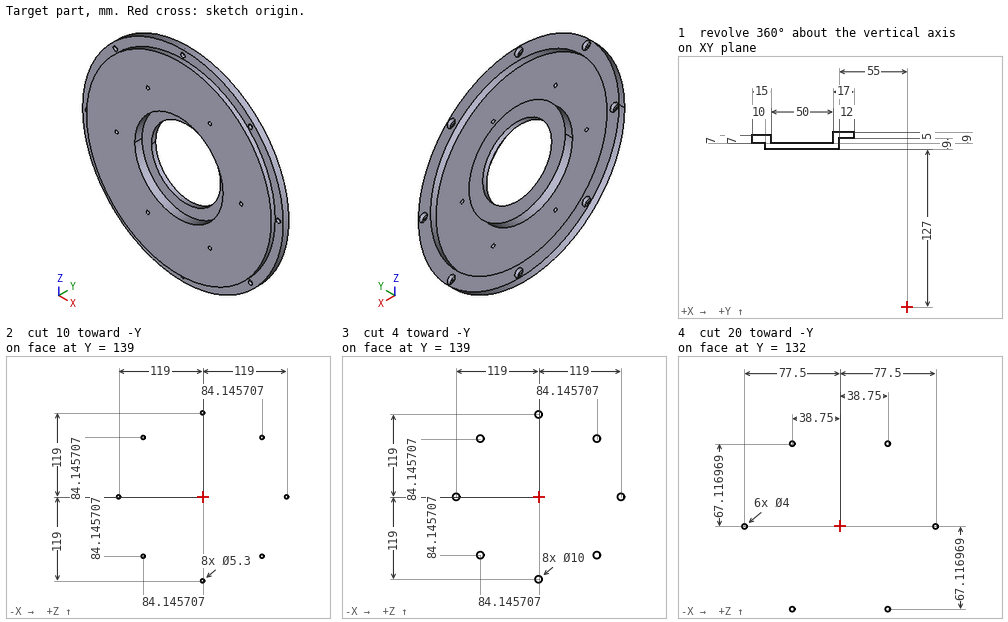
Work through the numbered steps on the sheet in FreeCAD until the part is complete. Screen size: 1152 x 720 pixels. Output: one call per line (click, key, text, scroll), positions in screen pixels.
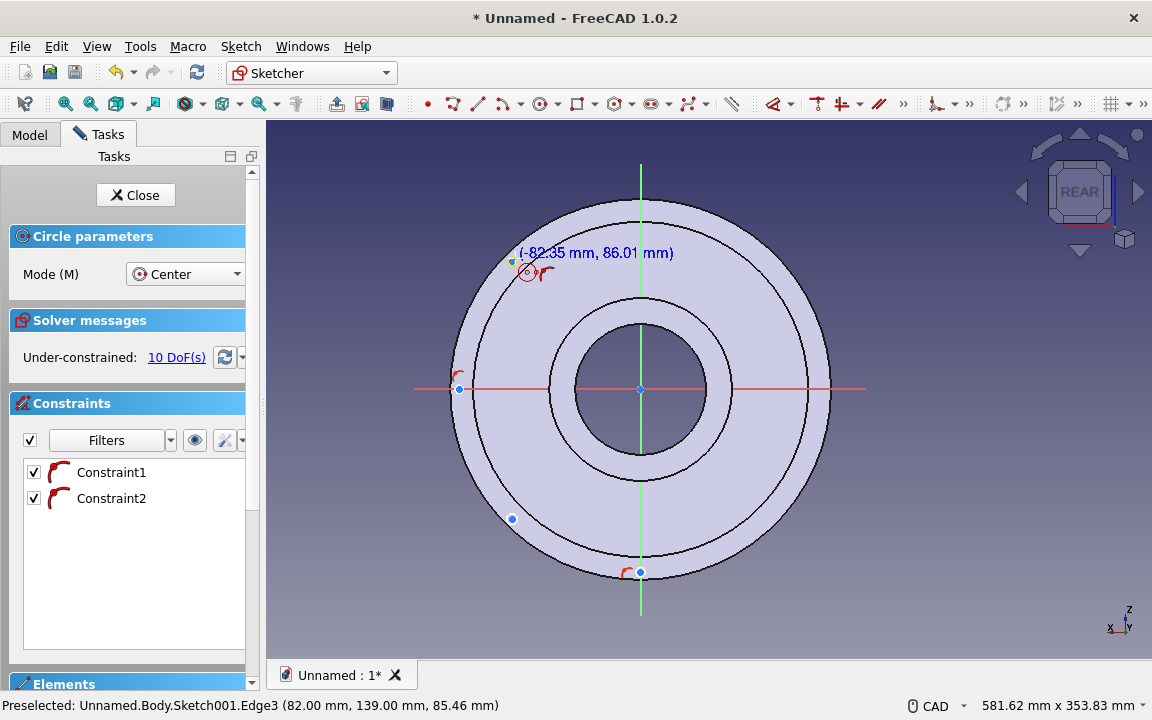
scroll(641, 208, up, 9)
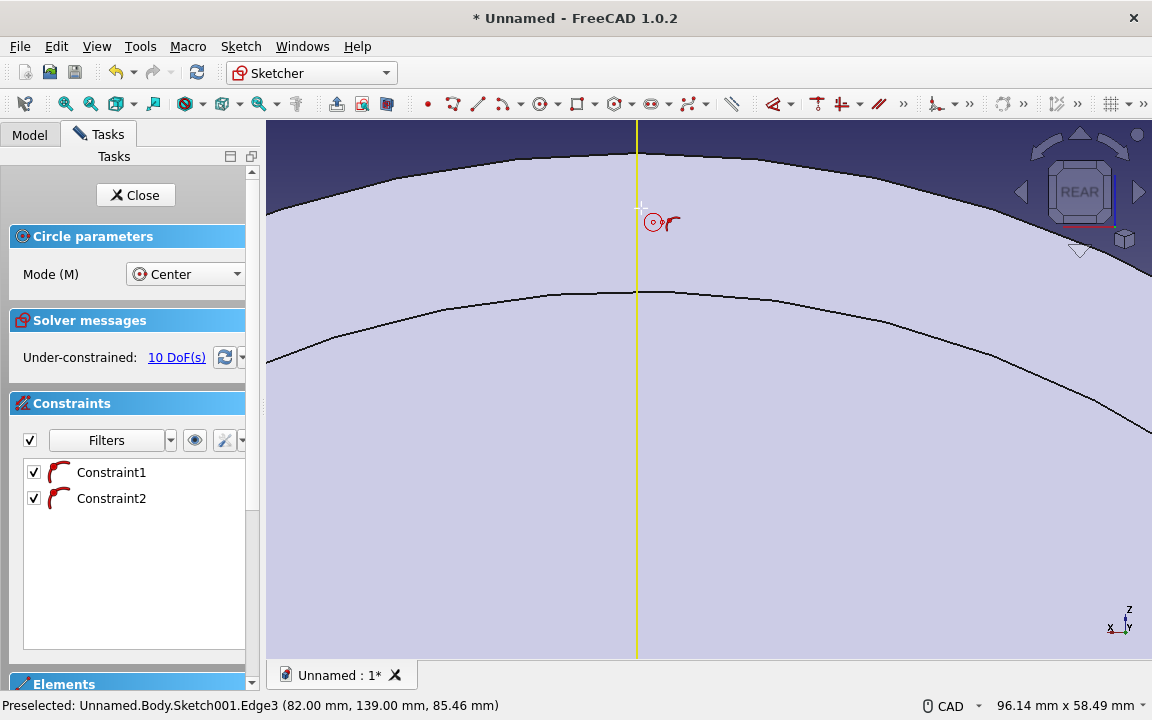
scroll(641, 208, down, 9)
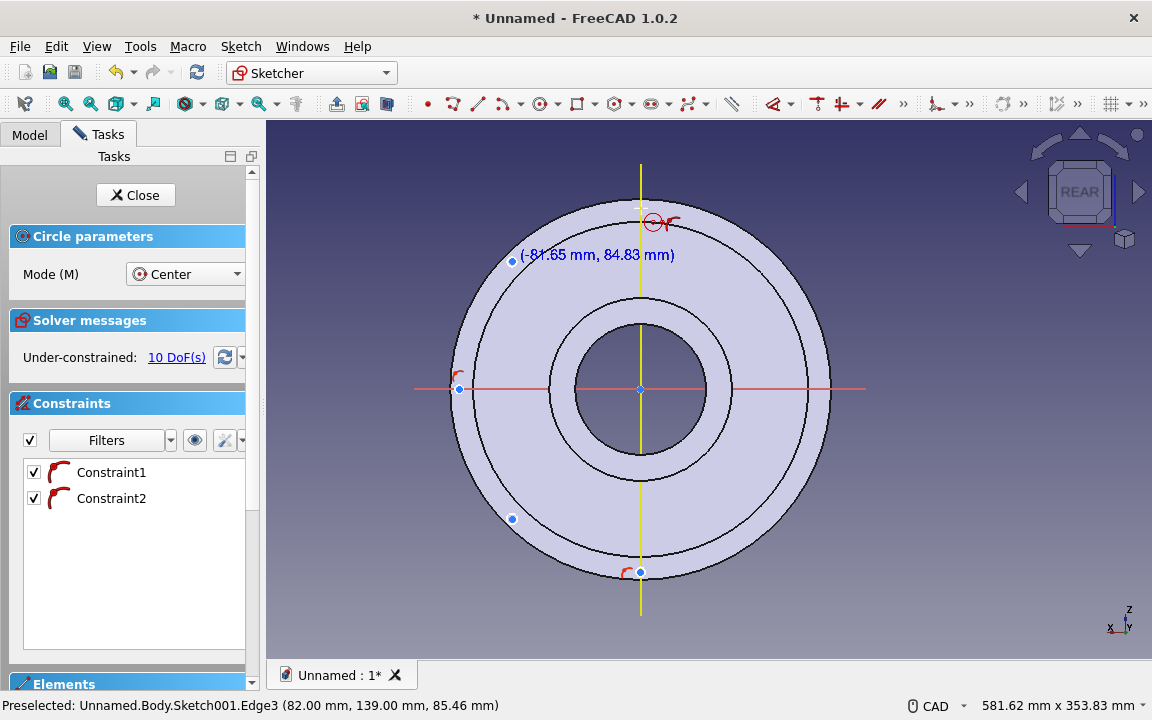
click(641, 208)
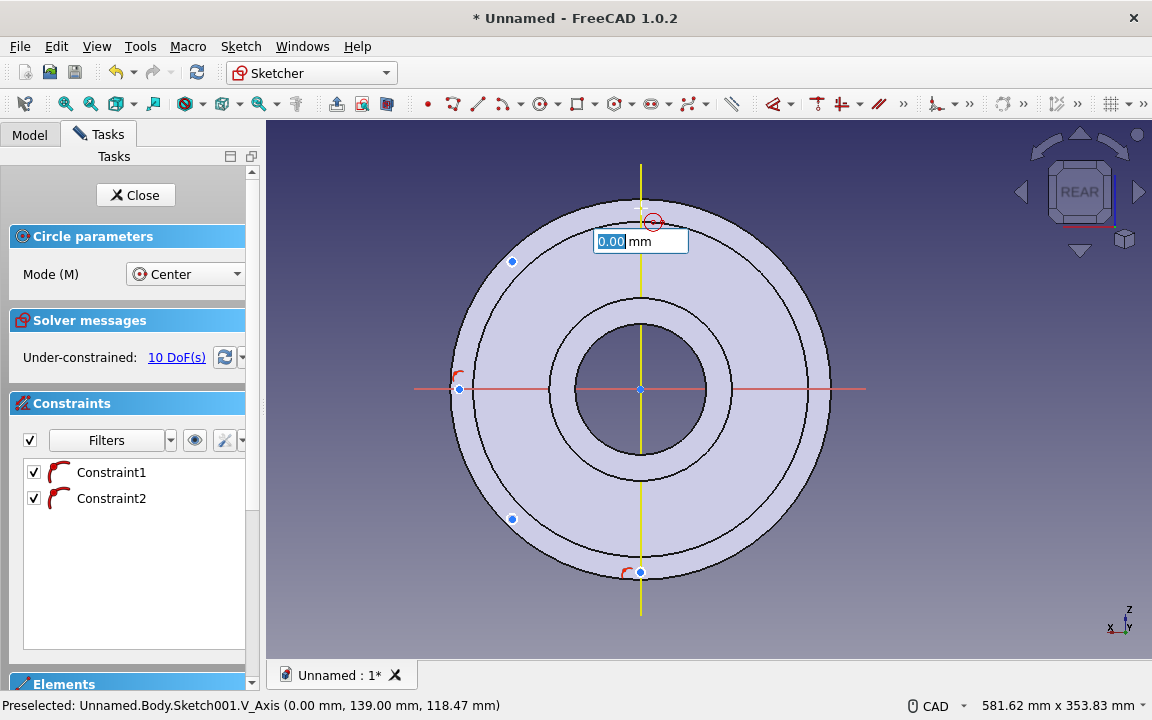
scroll(644, 207, up, 8)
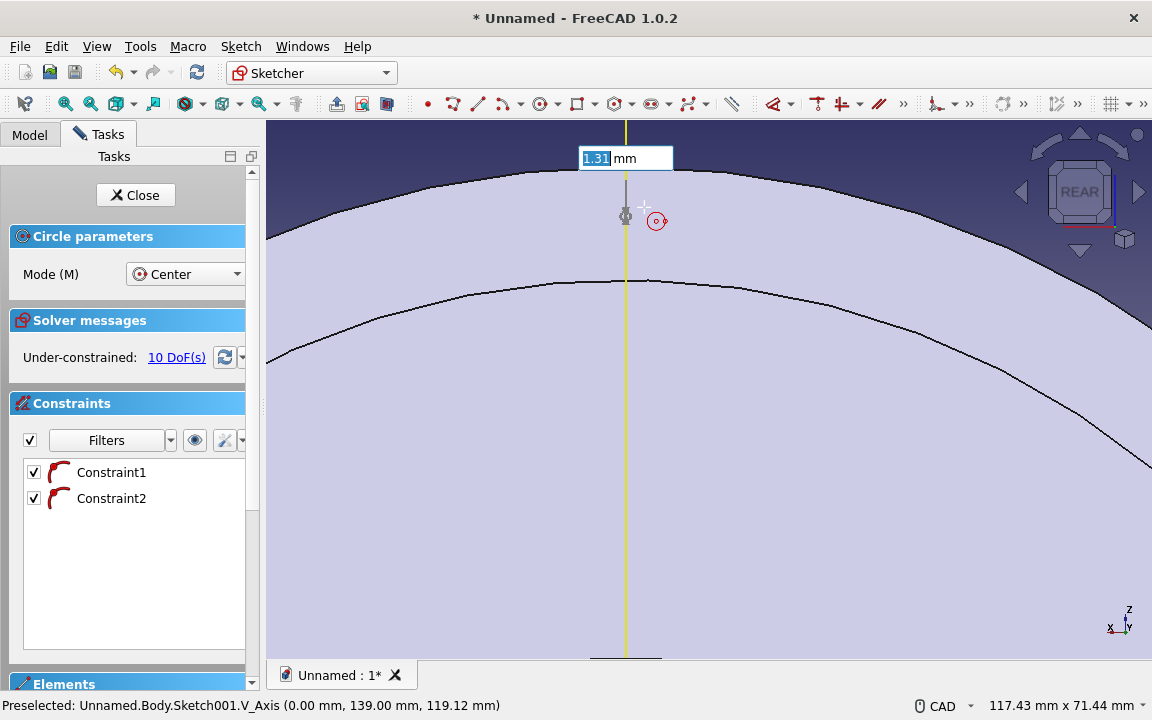
click(645, 205)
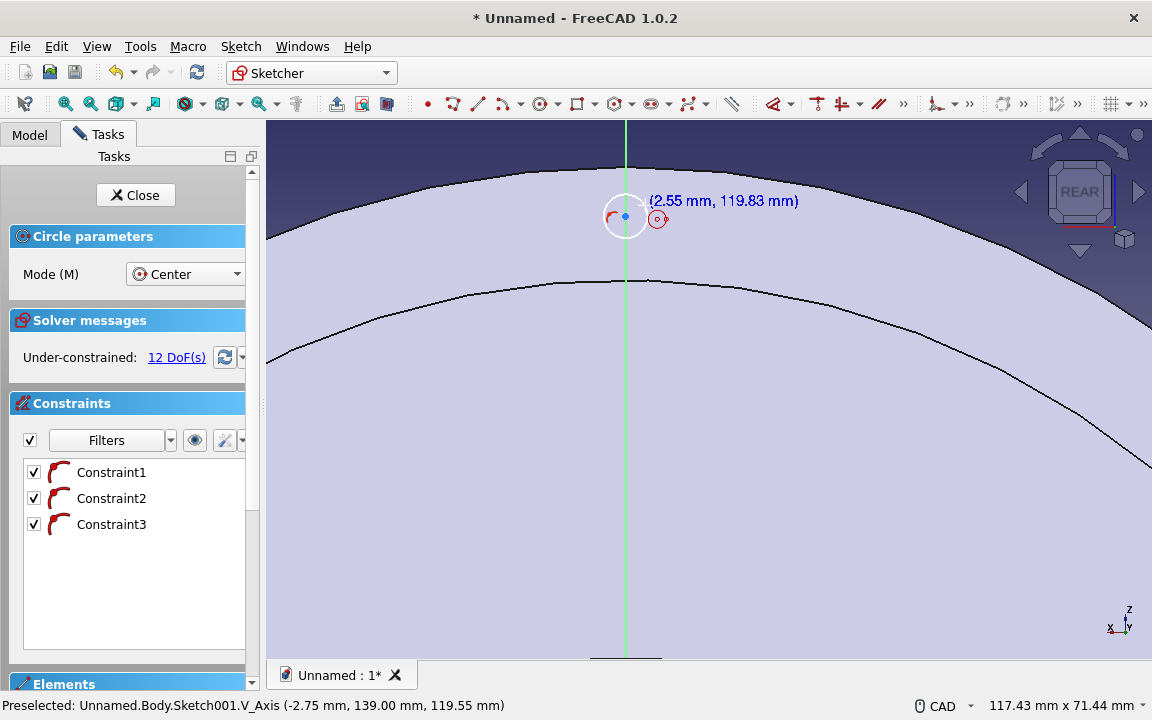
scroll(644, 207, down, 8)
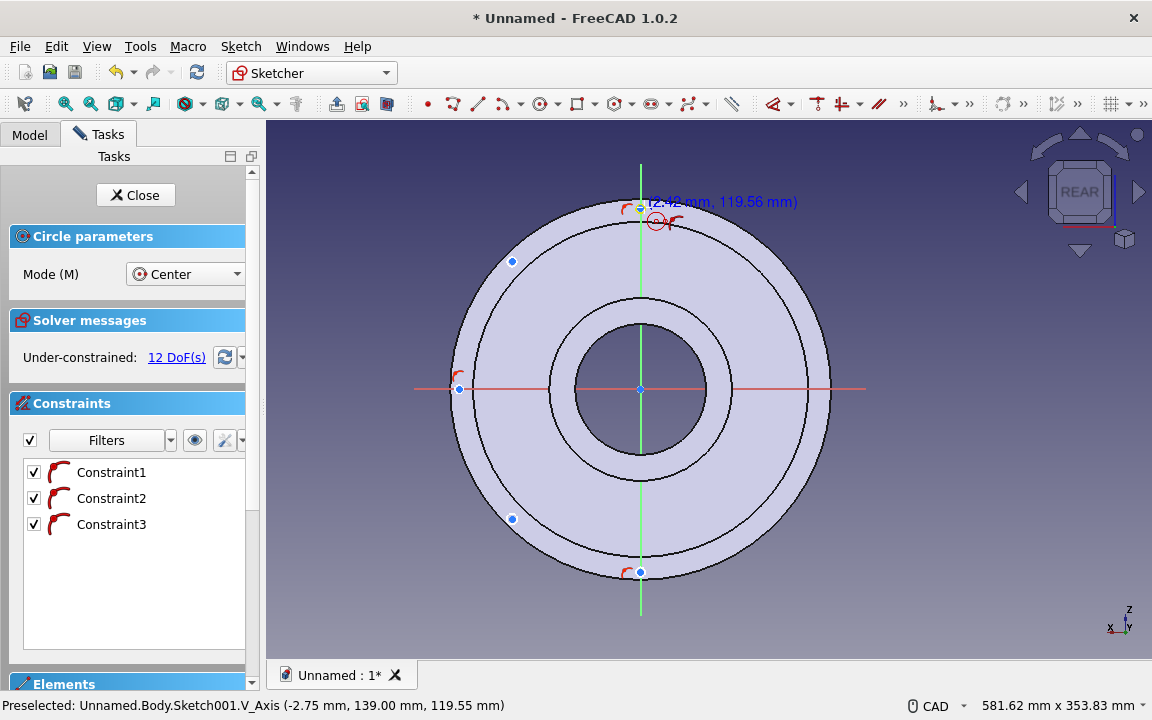
scroll(769, 261, up, 9)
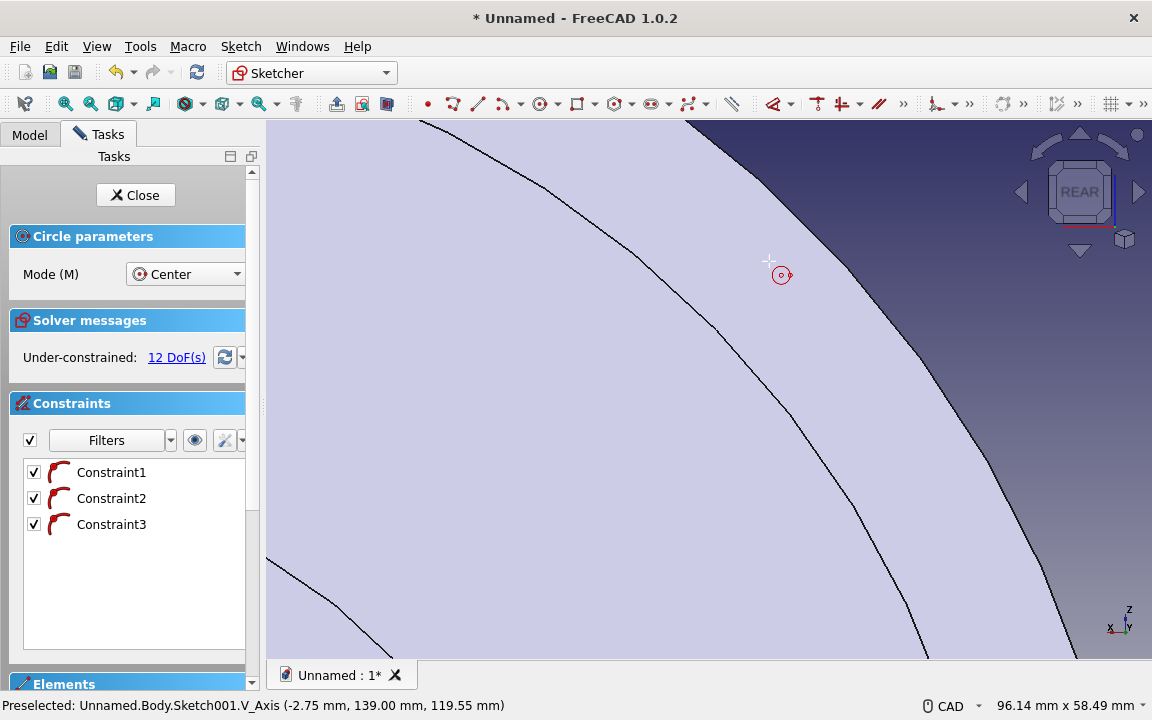
scroll(769, 261, down, 9)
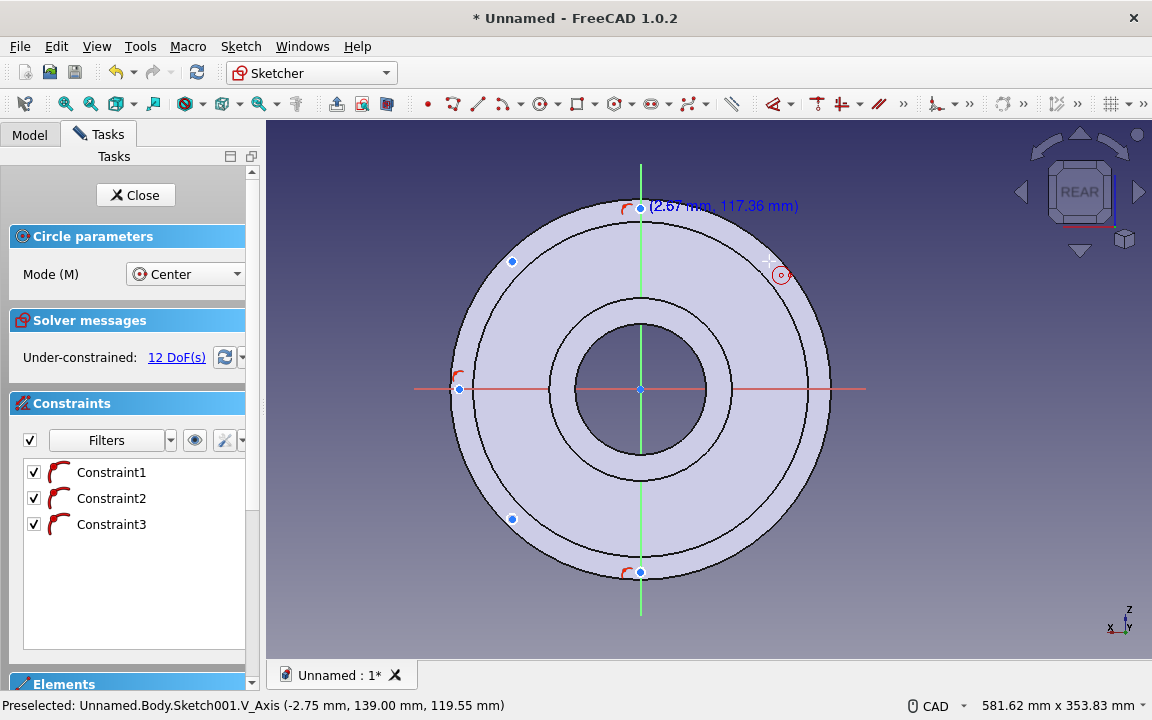
click(769, 261)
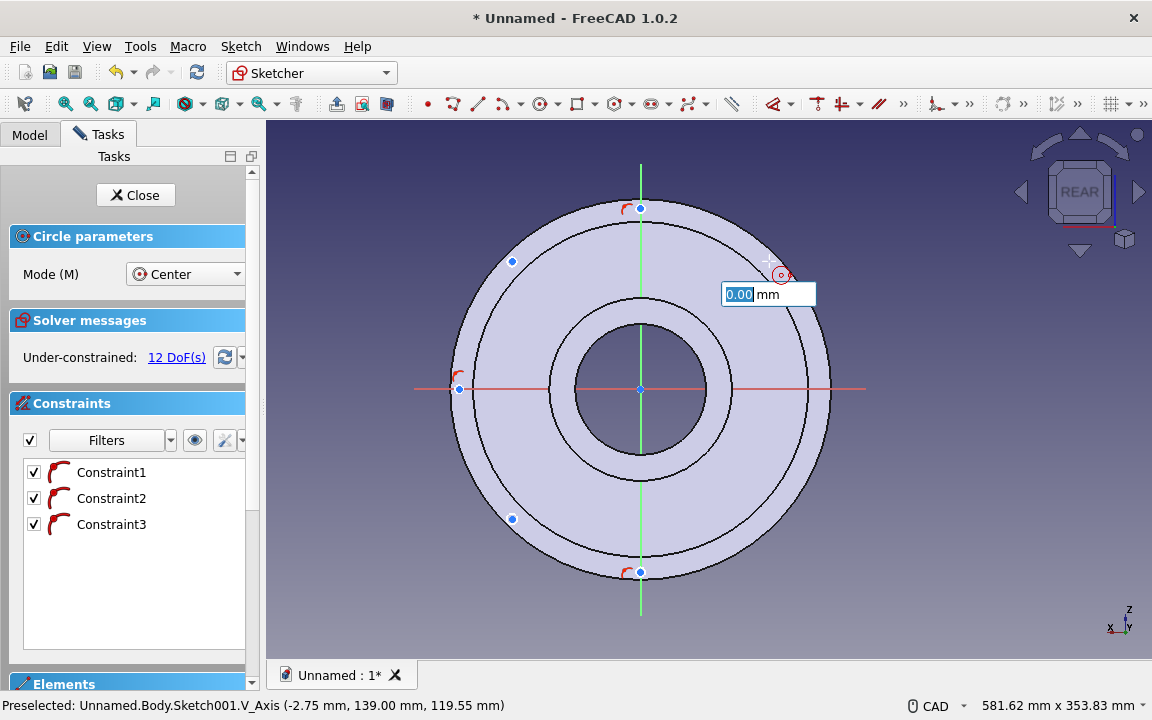
scroll(772, 258, up, 7)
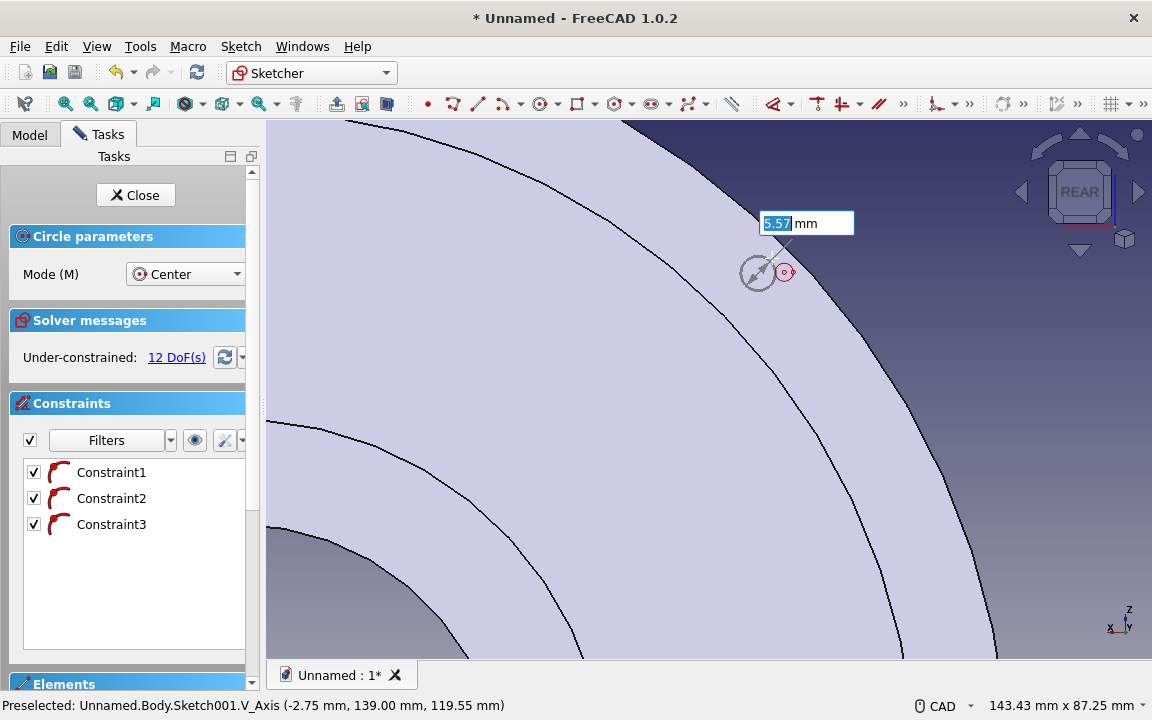
click(769, 259)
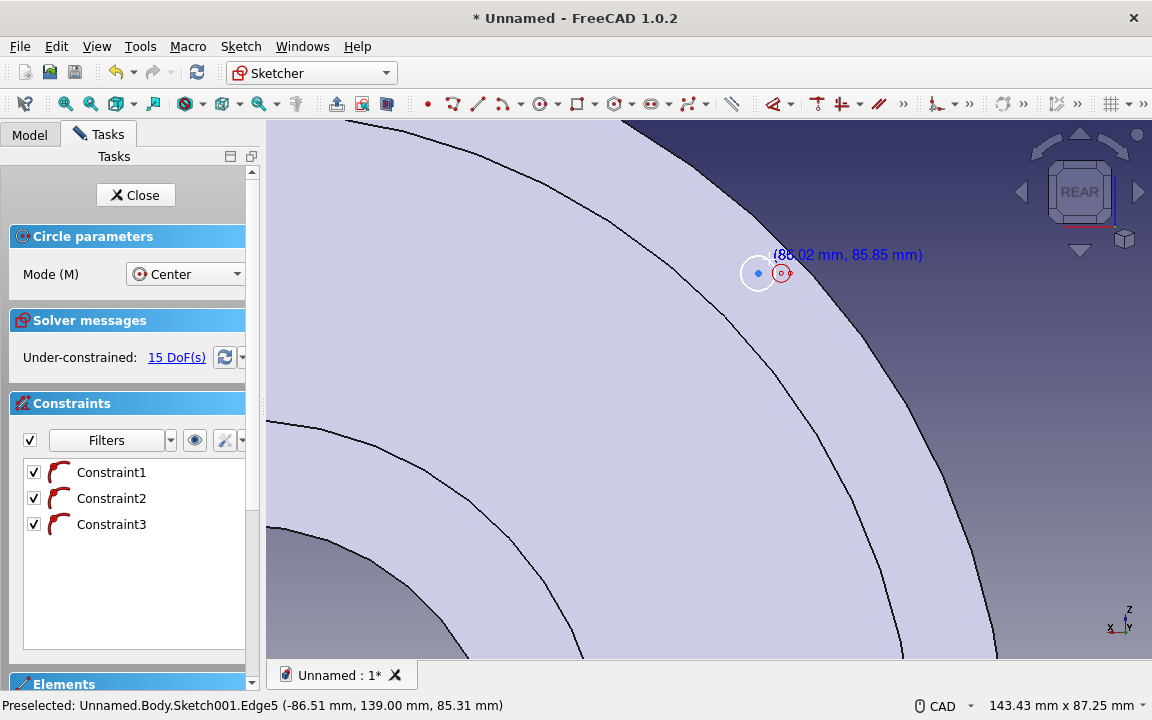
scroll(772, 258, down, 7)